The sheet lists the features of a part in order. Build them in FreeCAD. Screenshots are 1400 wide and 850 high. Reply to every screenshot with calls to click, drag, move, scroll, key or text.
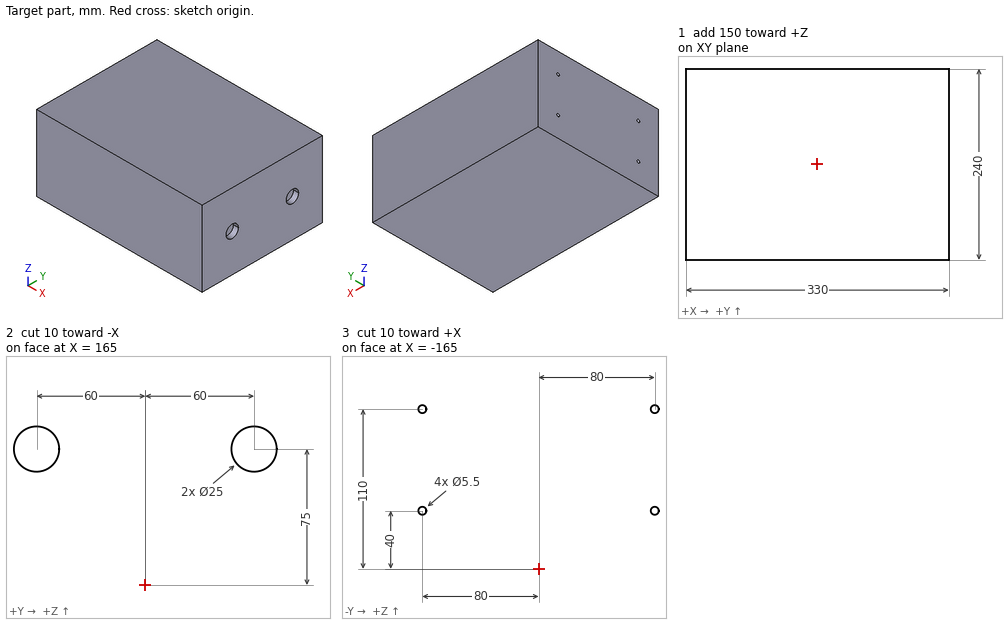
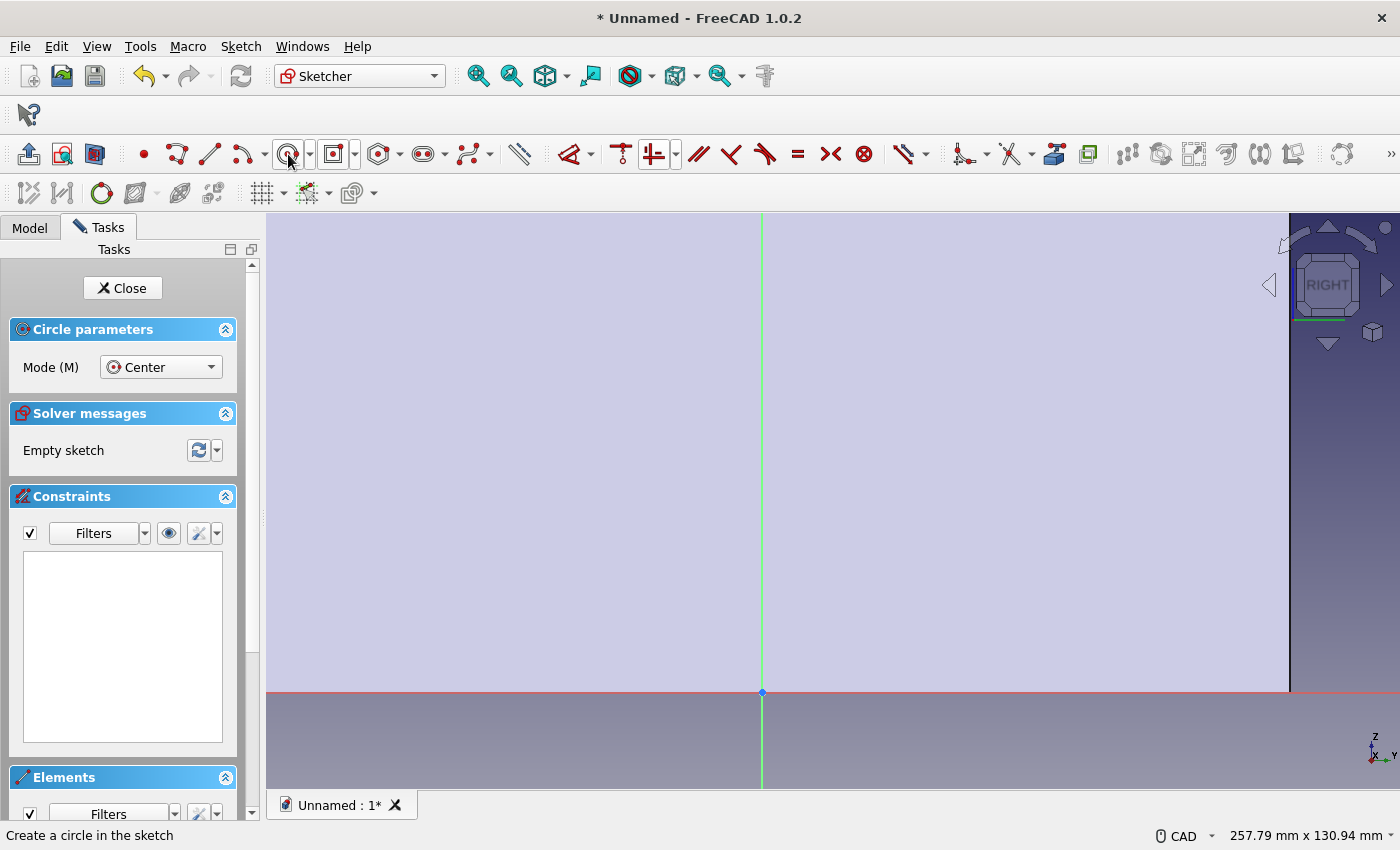
click(1026, 363)
move(1065, 324)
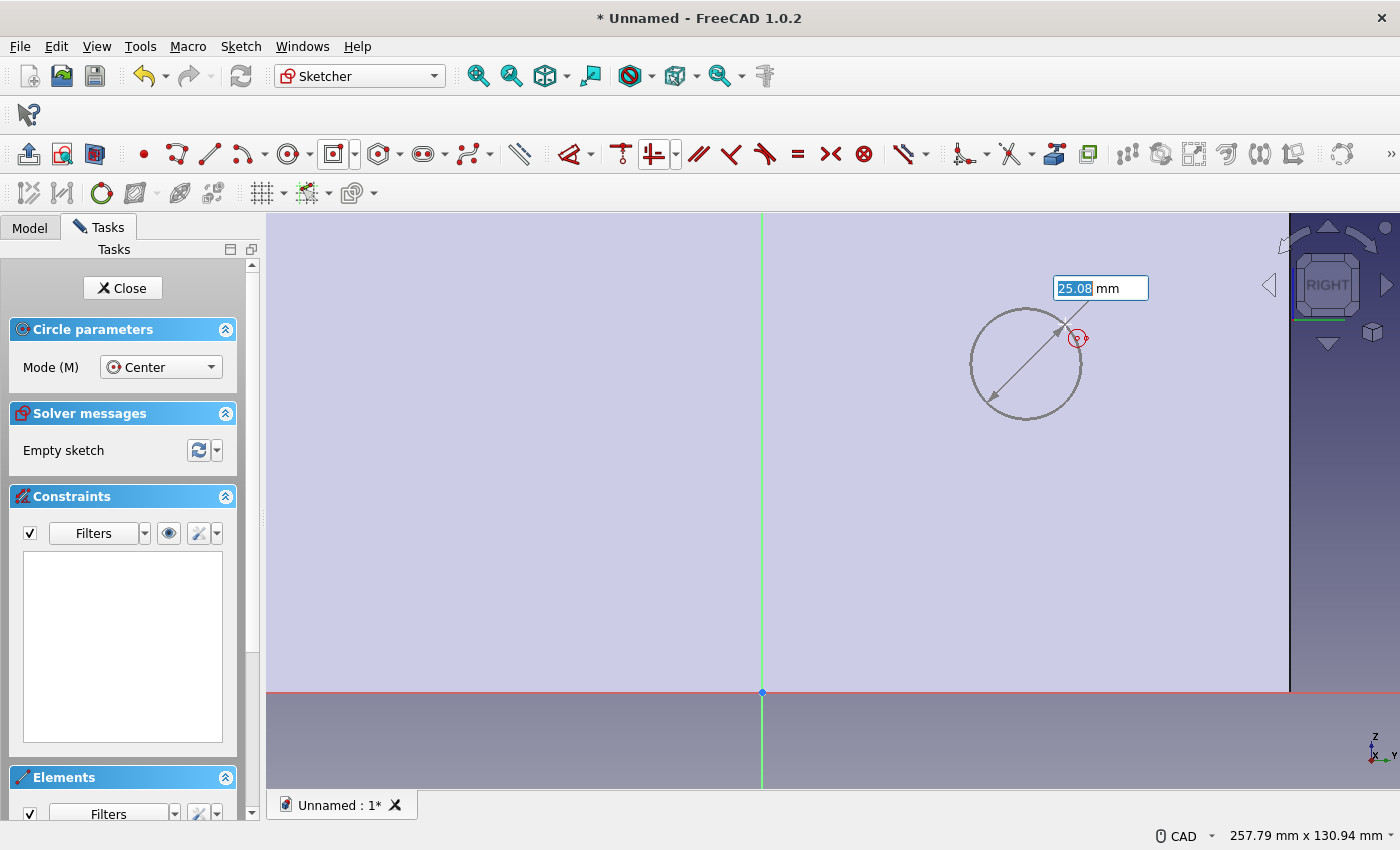
text(25)
key(Return)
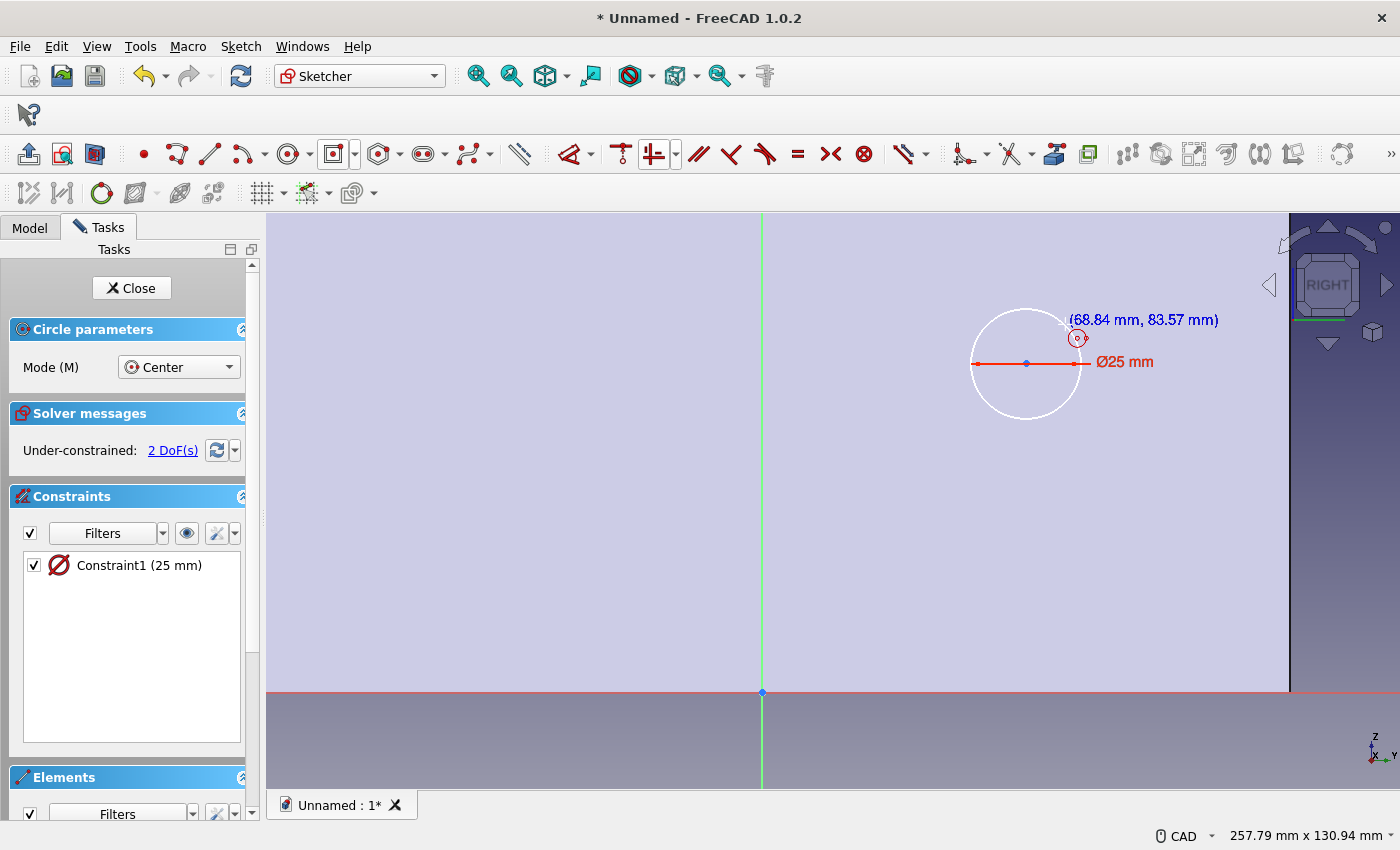
click(498, 363)
move(537, 324)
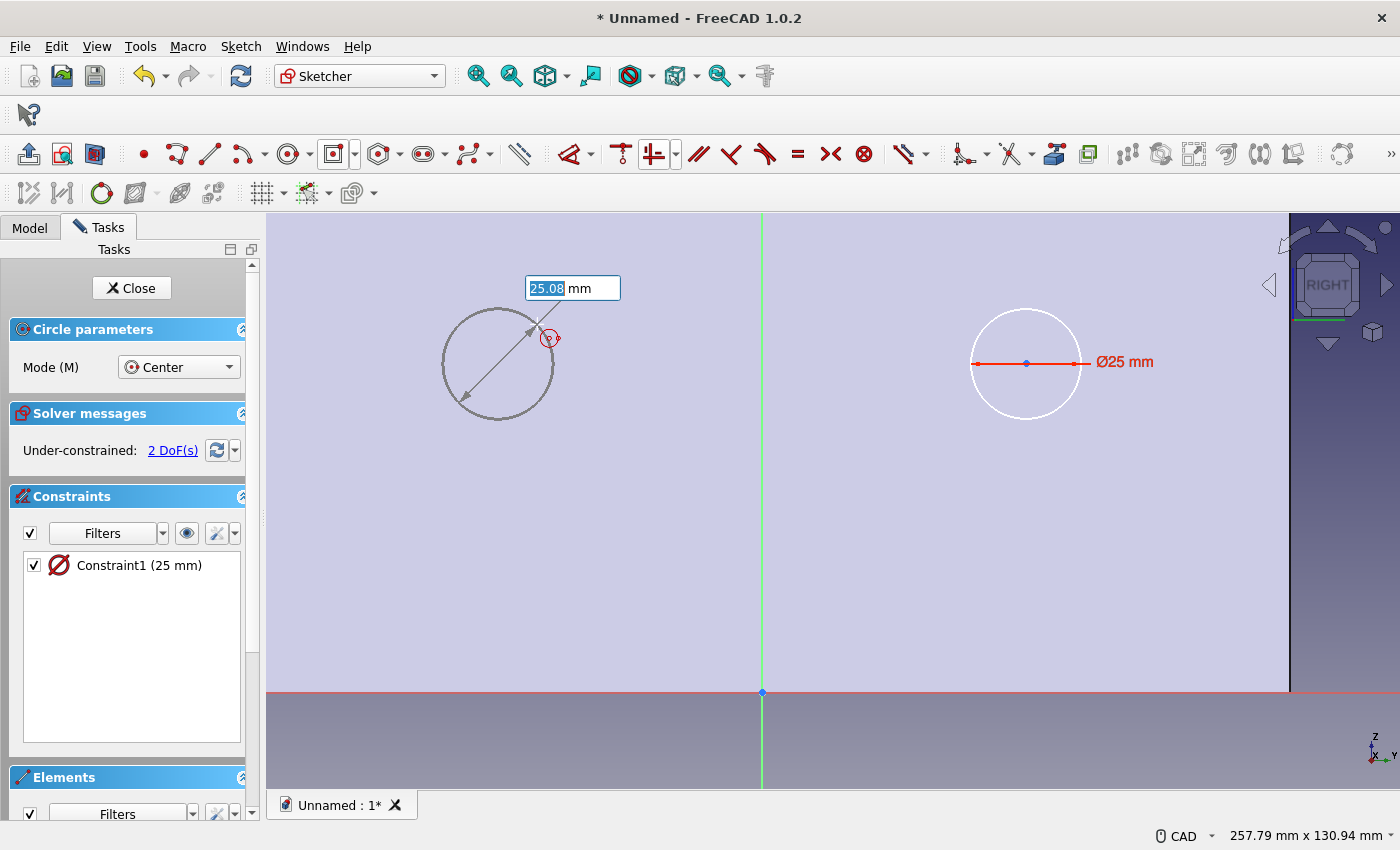
text(25)
key(Return)
key(Escape)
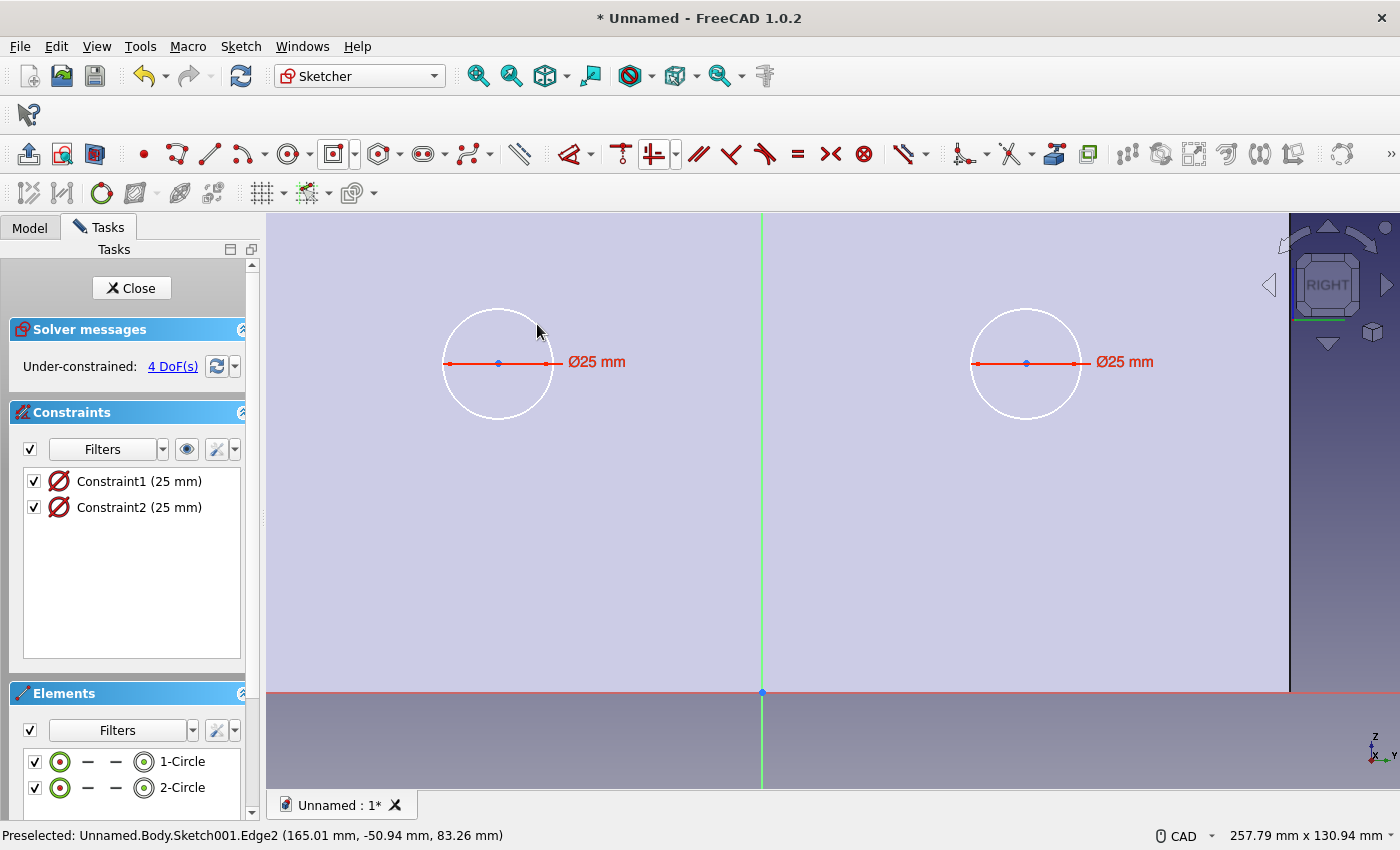
click(1026, 364)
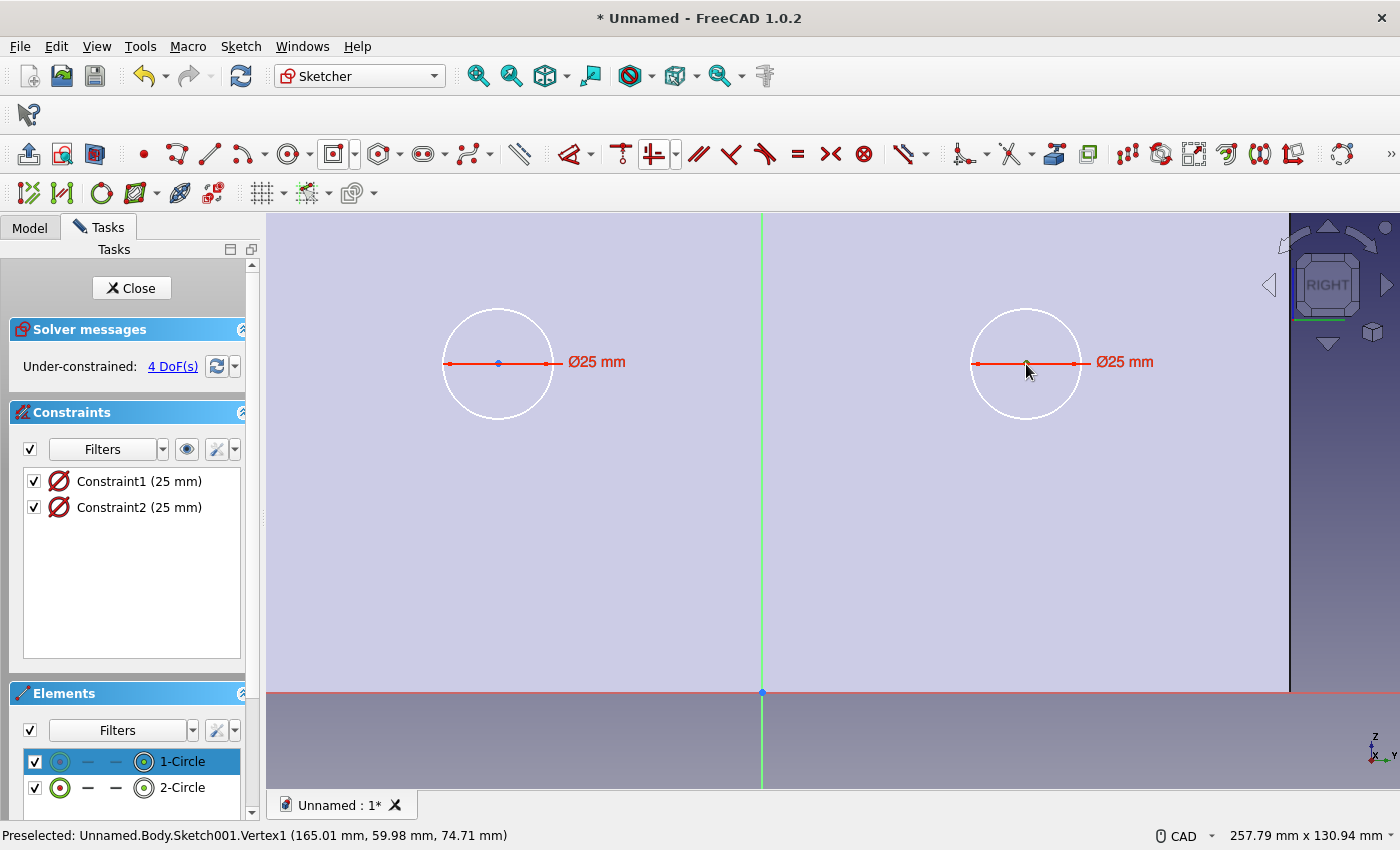
click(498, 364)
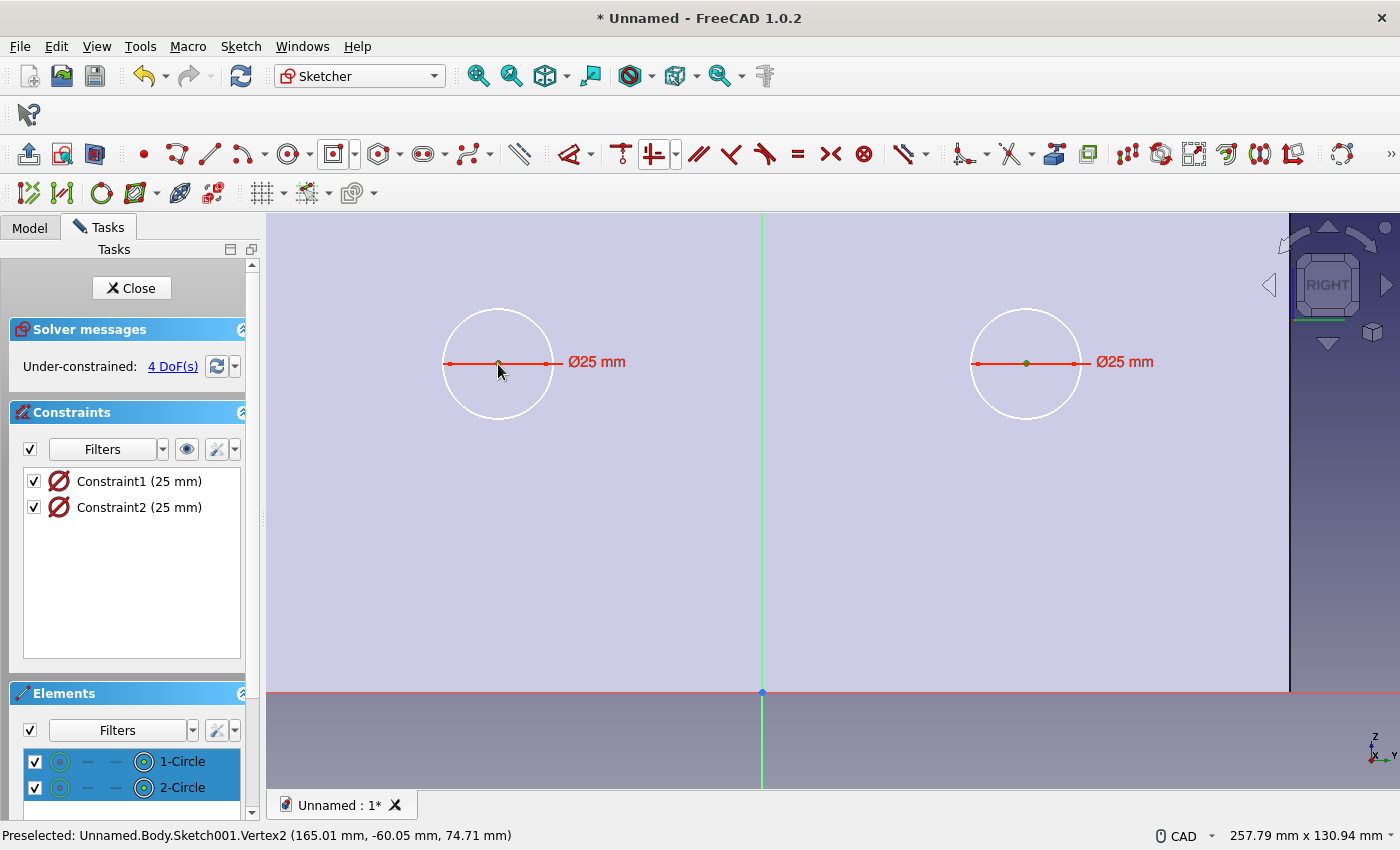
key(h)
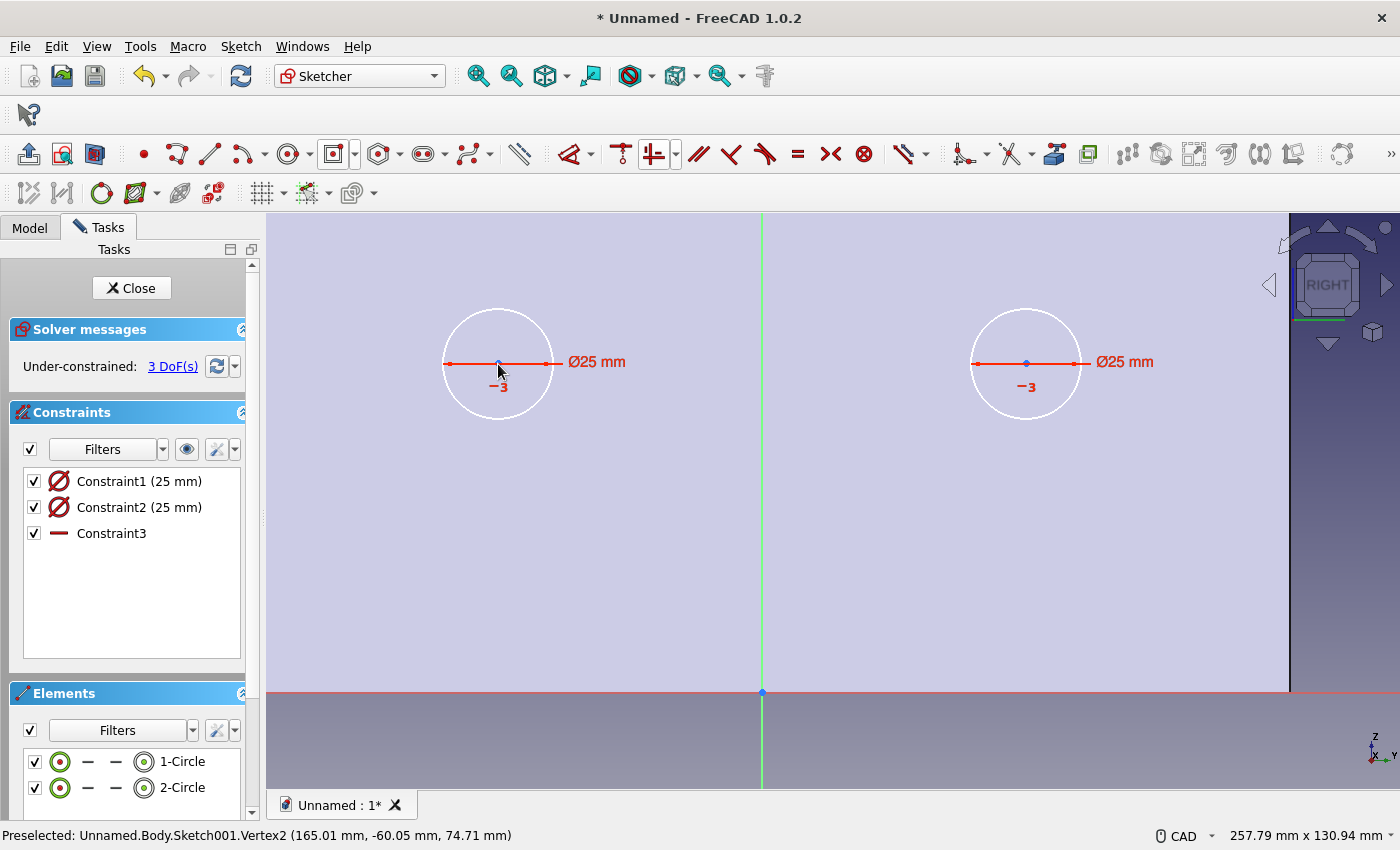
click(568, 154)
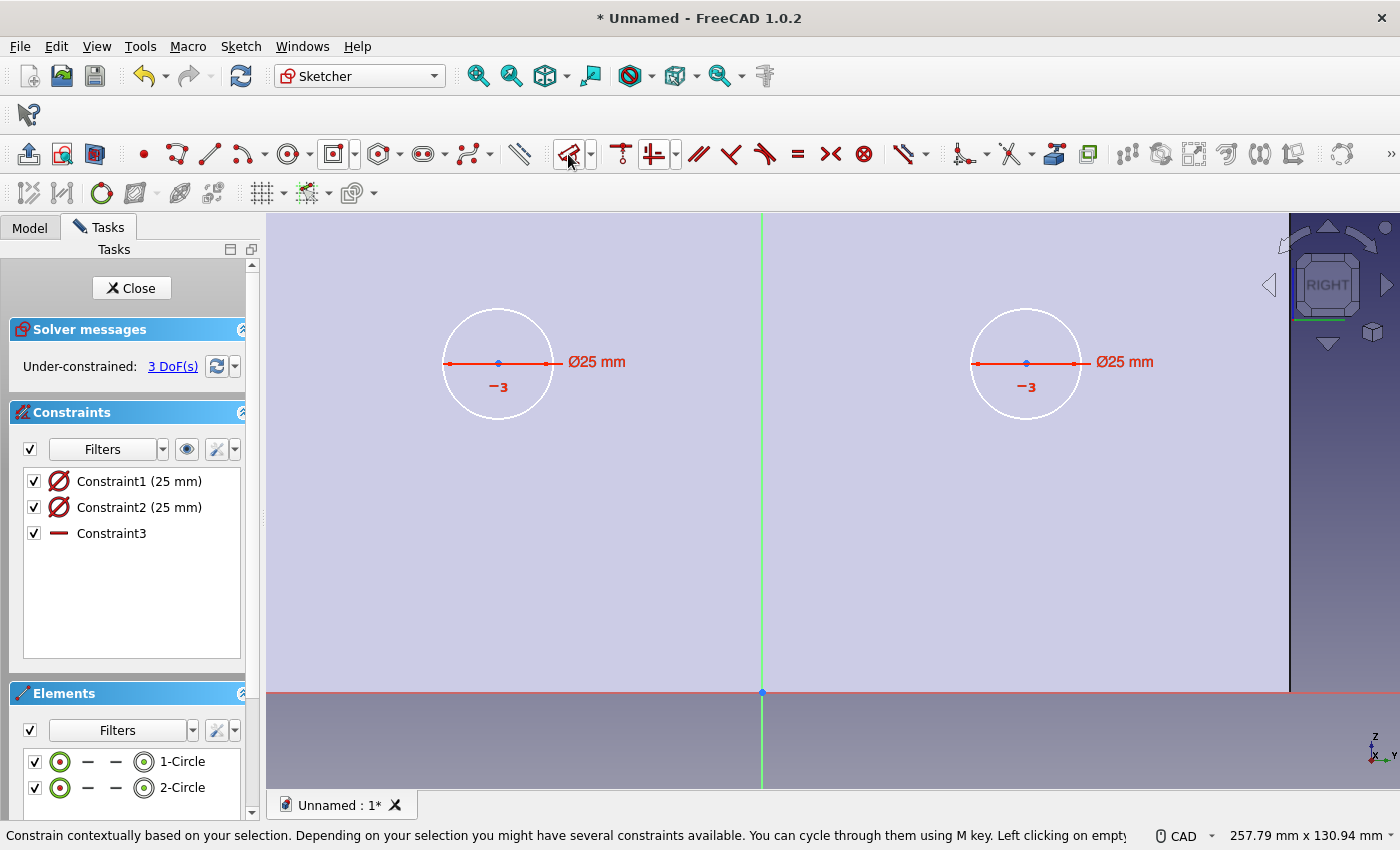
click(1026, 364)
click(894, 727)